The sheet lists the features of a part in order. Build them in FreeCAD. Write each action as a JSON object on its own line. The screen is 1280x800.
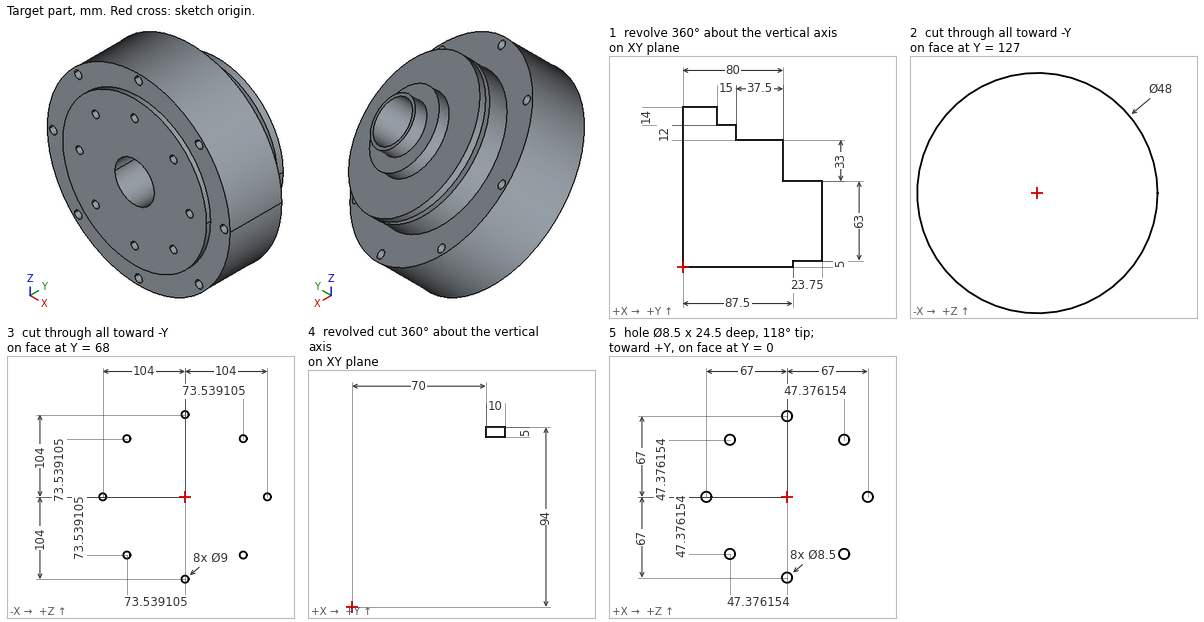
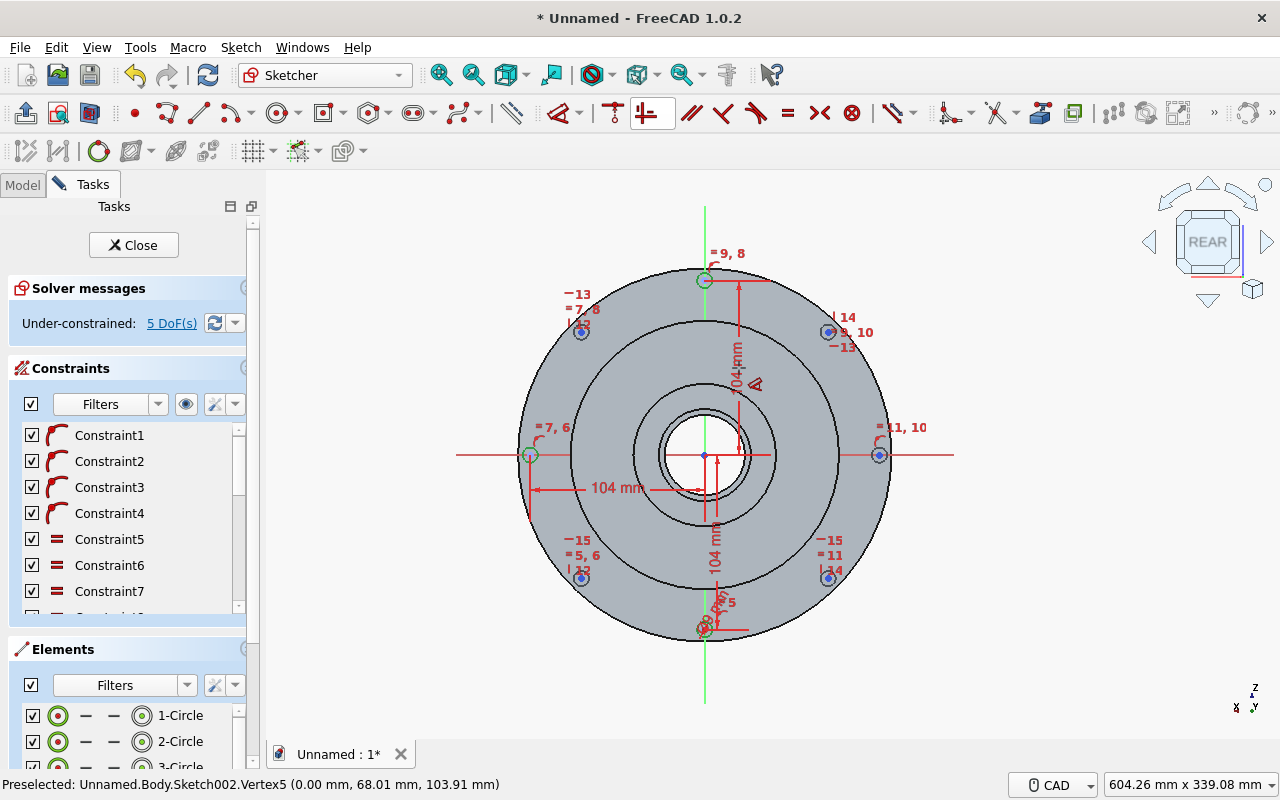
{"action": "left_click", "coordinate": [879, 455]}
{"action": "left_click", "coordinate": [792, 489]}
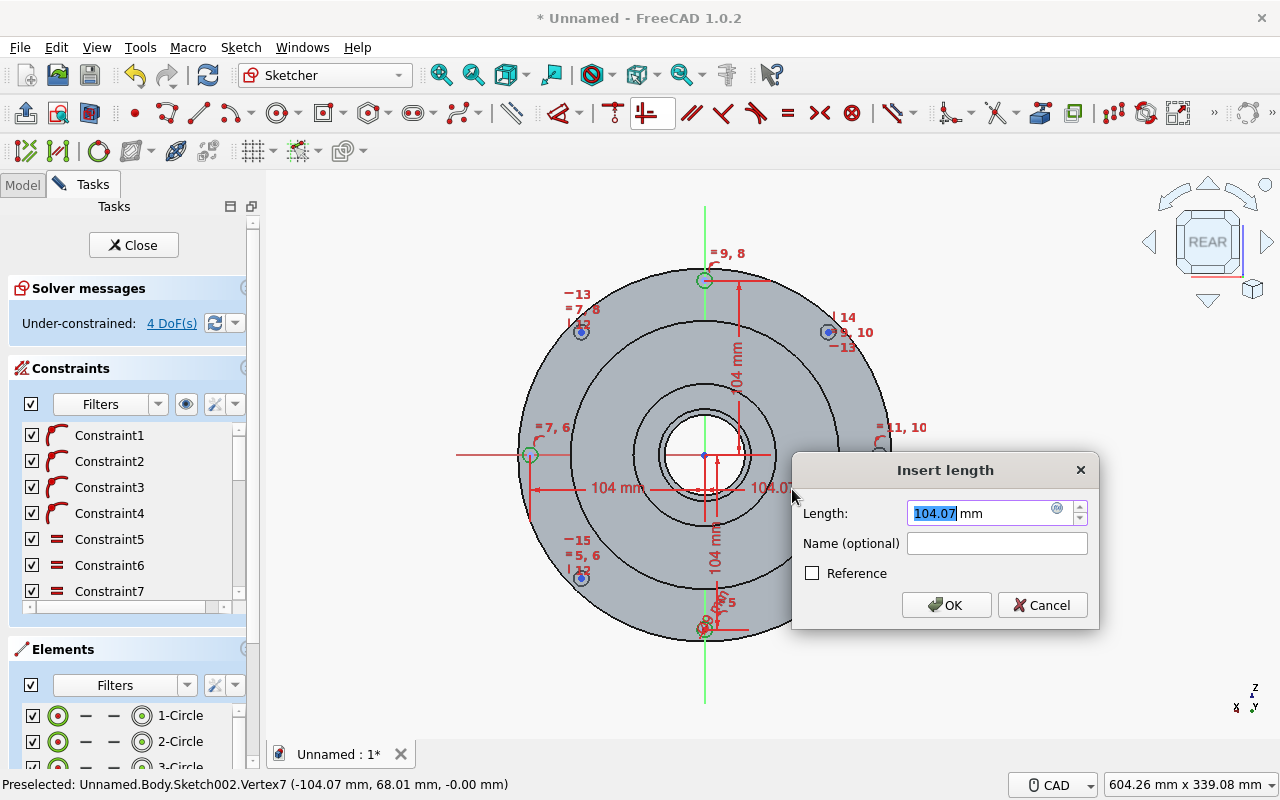
{"action": "type", "text": "104"}
{"action": "key", "text": "Return"}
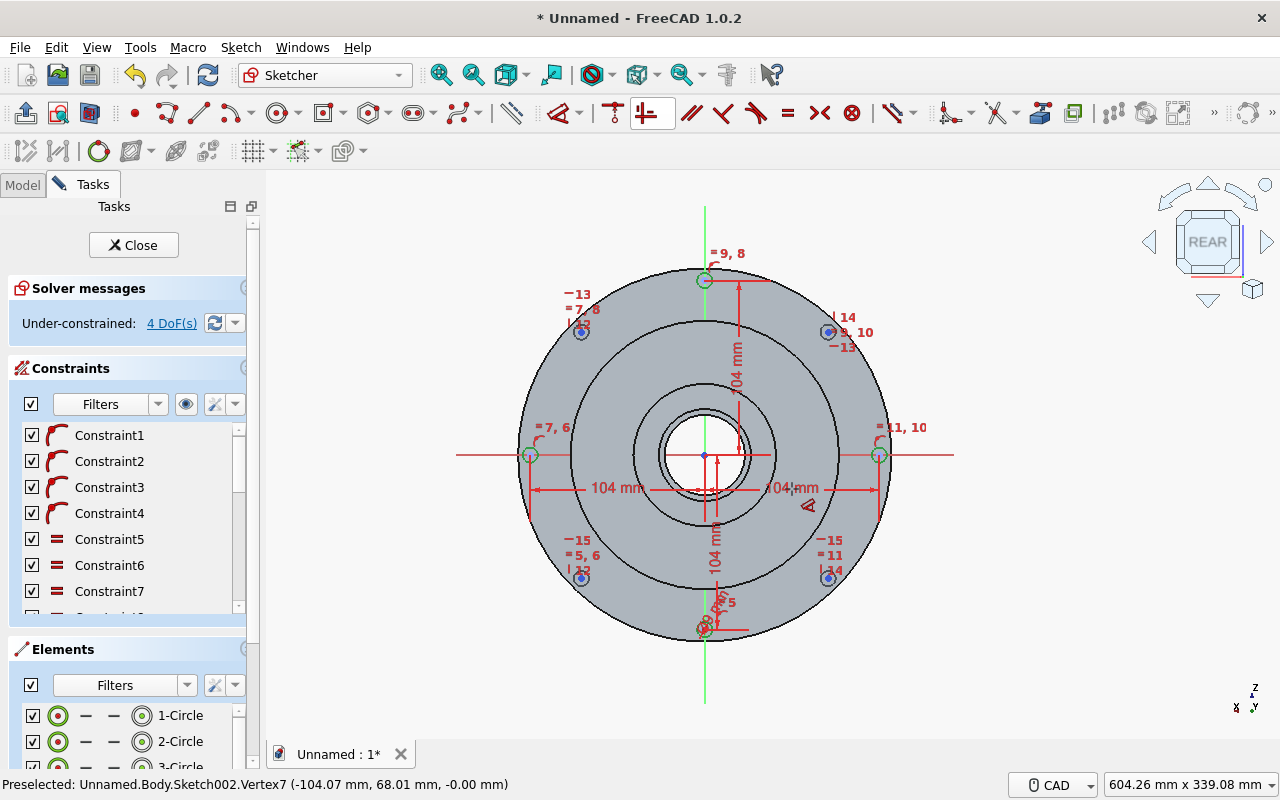
{"action": "left_click", "coordinate": [581, 579]}
{"action": "left_click", "coordinate": [643, 613]}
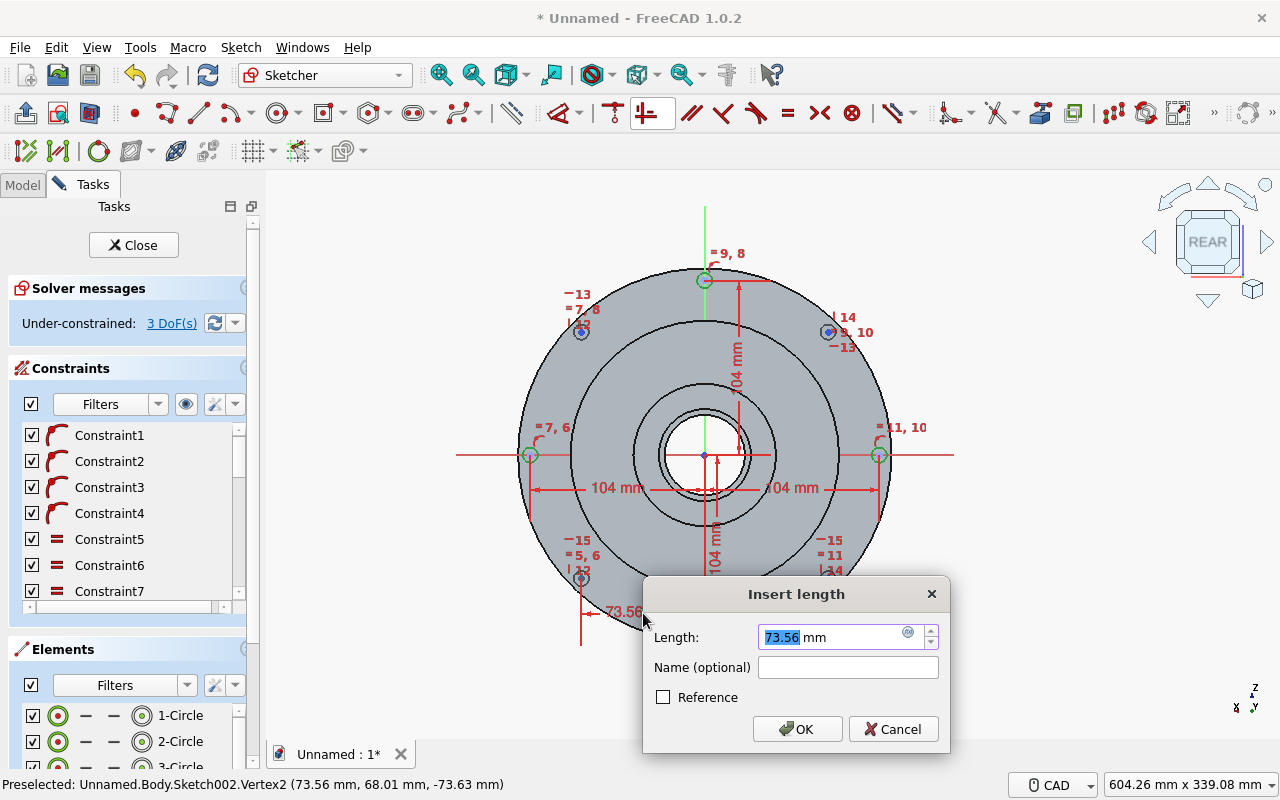
{"action": "type", "text": "73.539105"}
{"action": "key", "text": "Return"}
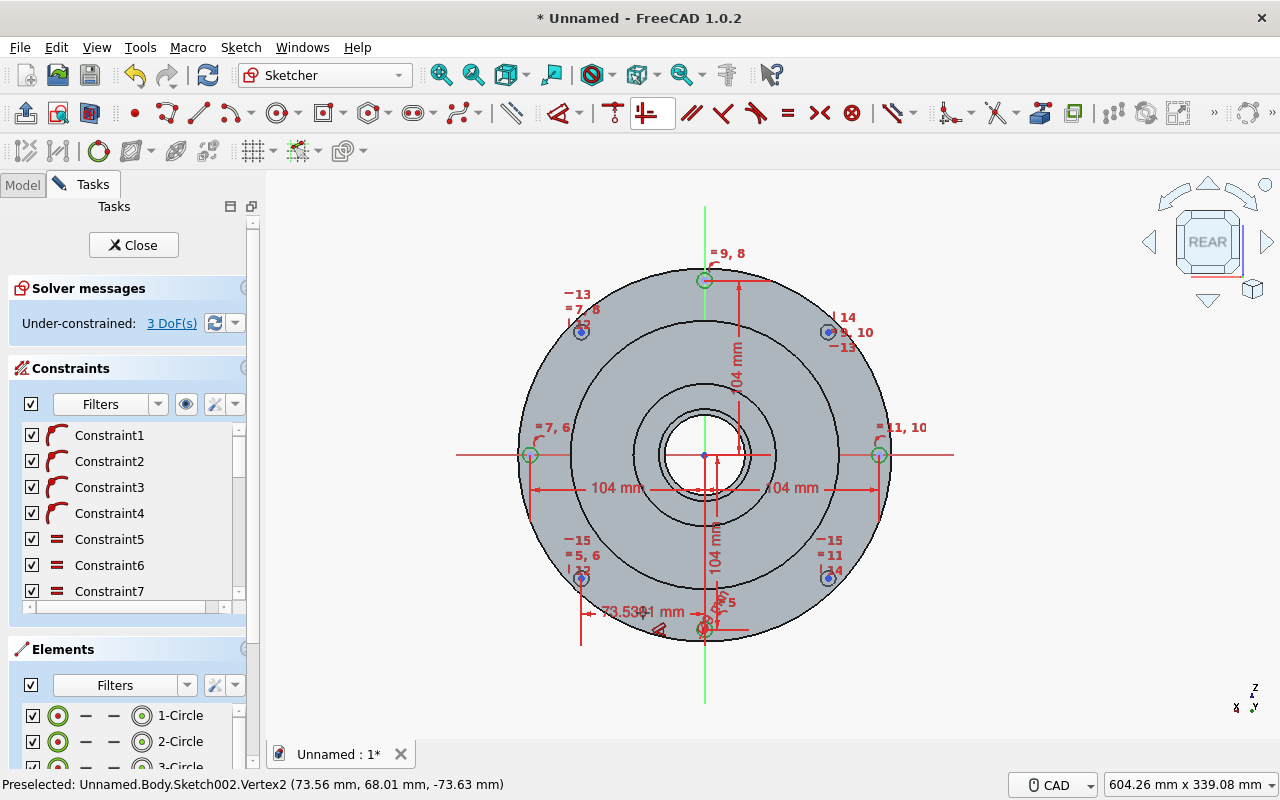
{"action": "left_click", "coordinate": [581, 579]}
{"action": "left_click", "coordinate": [547, 517]}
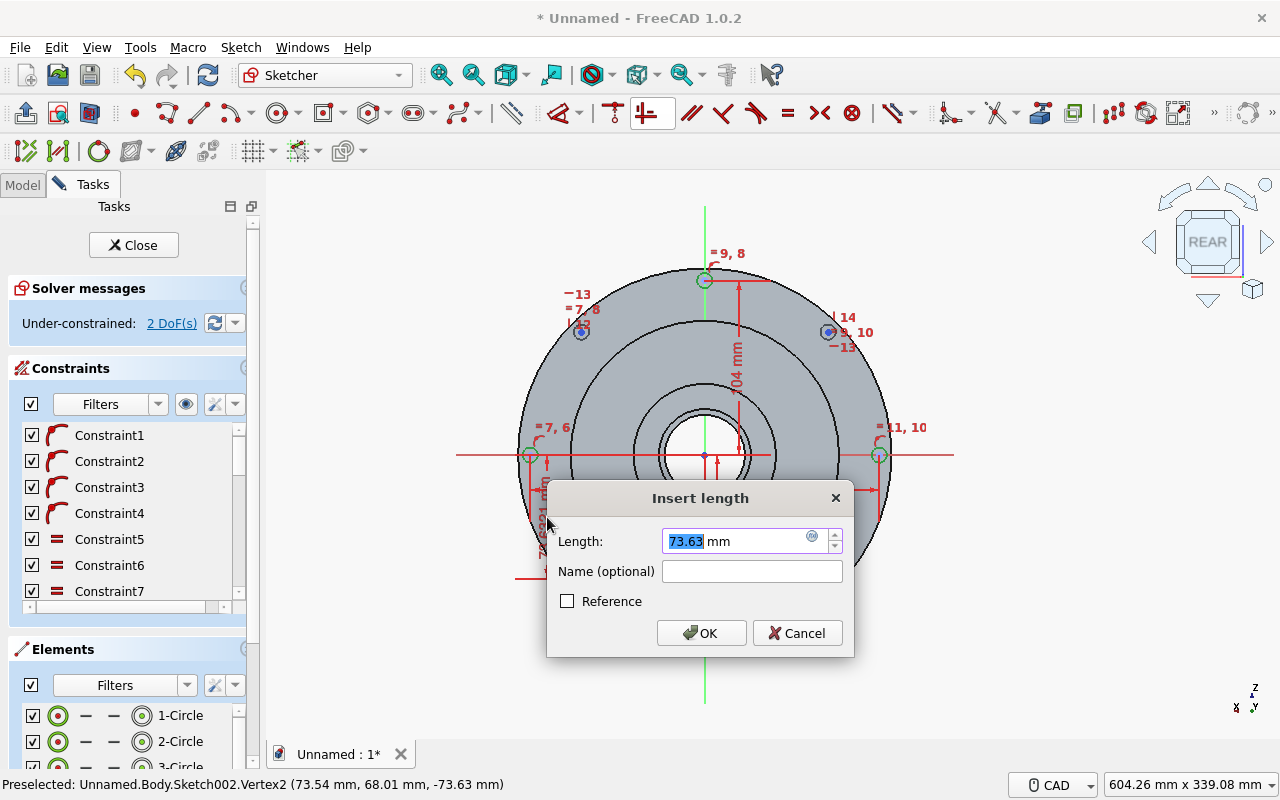
{"action": "type", "text": "73.539105"}
{"action": "key", "text": "Return"}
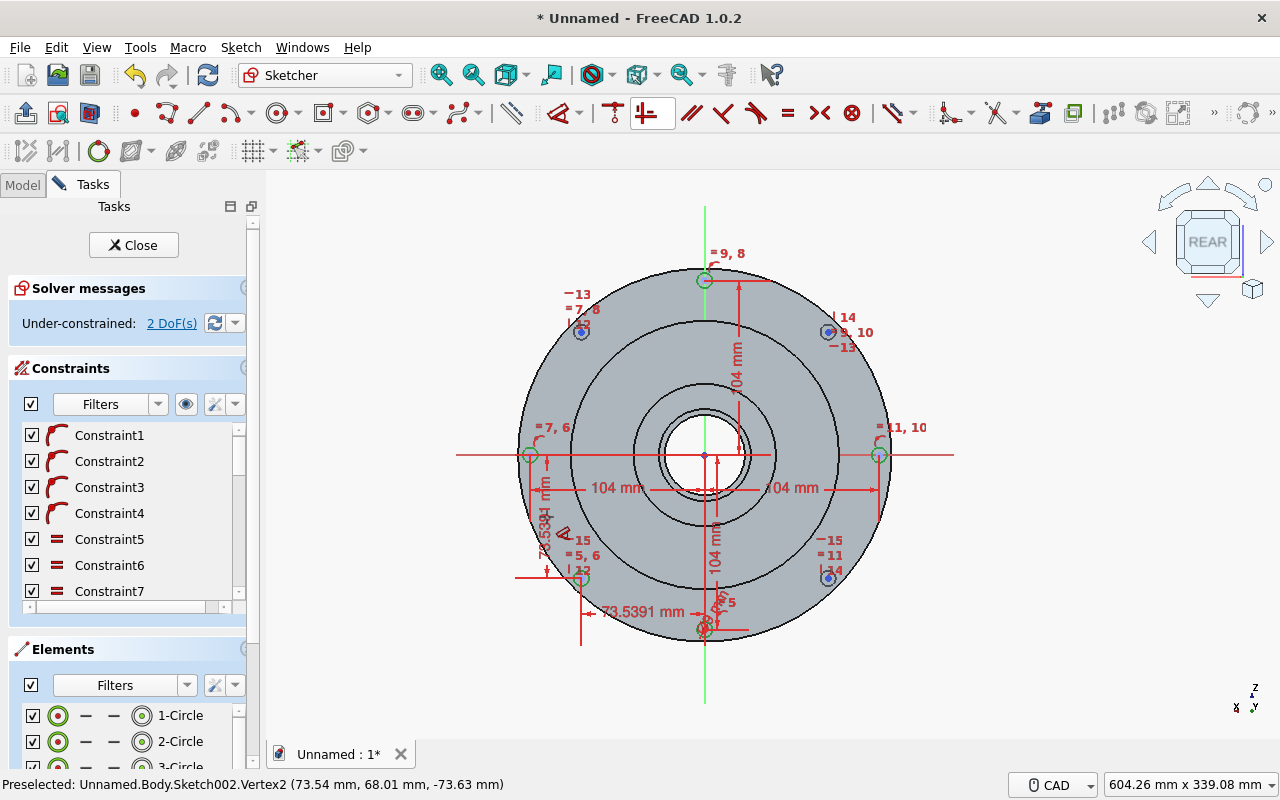
{"action": "left_click", "coordinate": [581, 332]}
{"action": "left_click", "coordinate": [547, 394]}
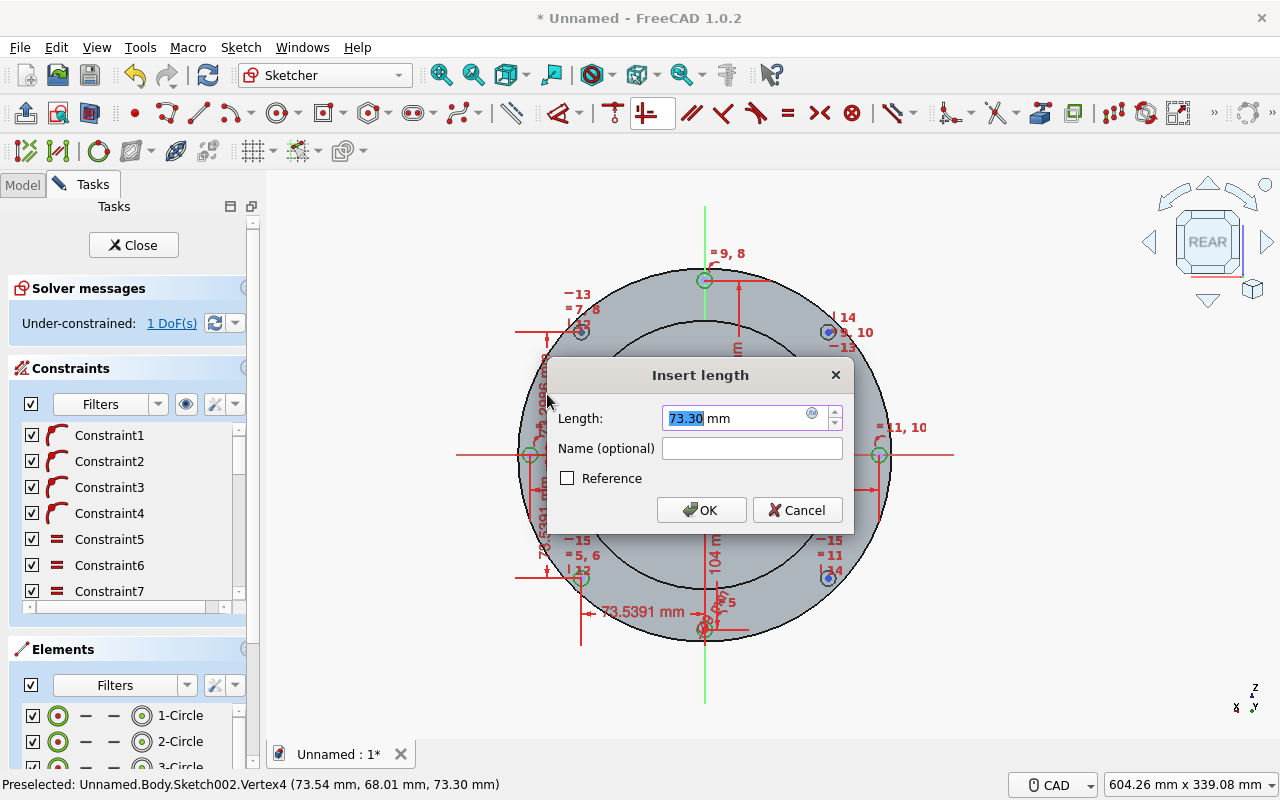
{"action": "type", "text": "73.539105"}
{"action": "key", "text": "Return"}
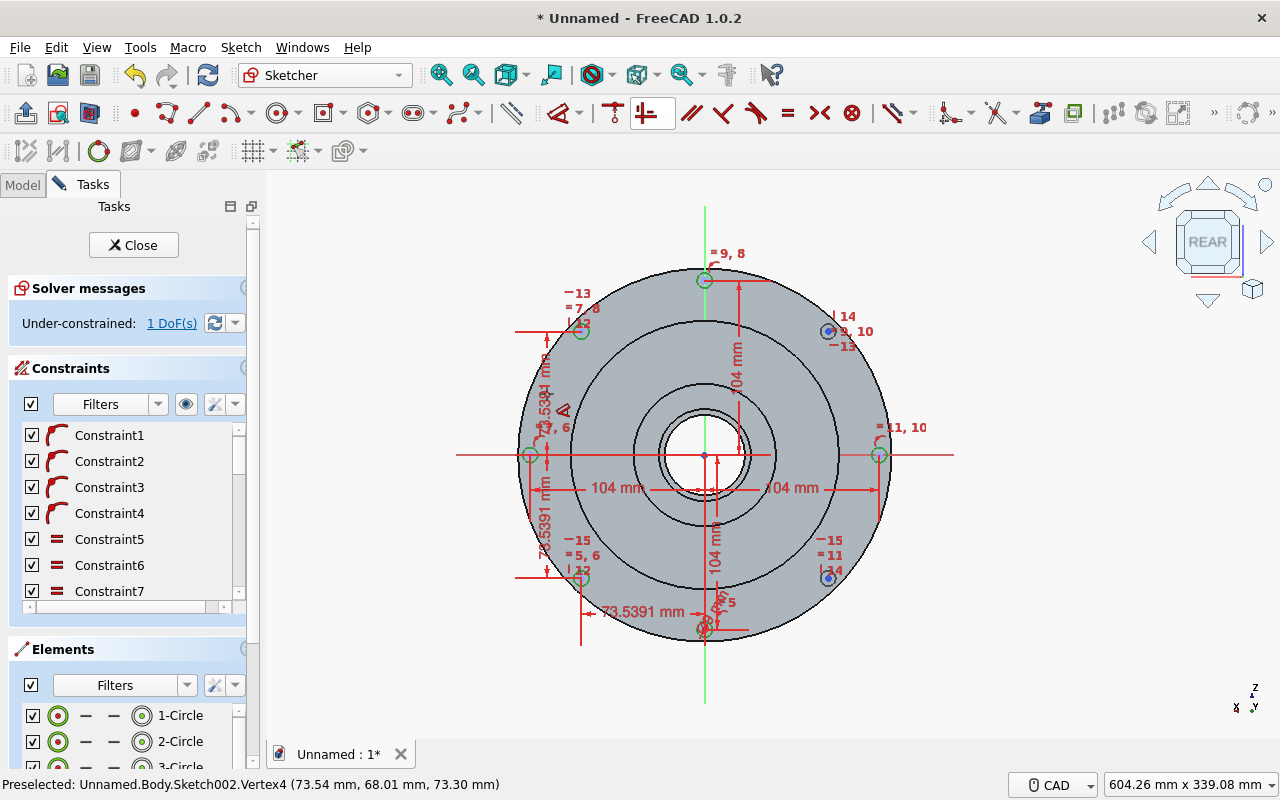
{"action": "left_click", "coordinate": [828, 332]}
{"action": "left_click", "coordinate": [766, 298]}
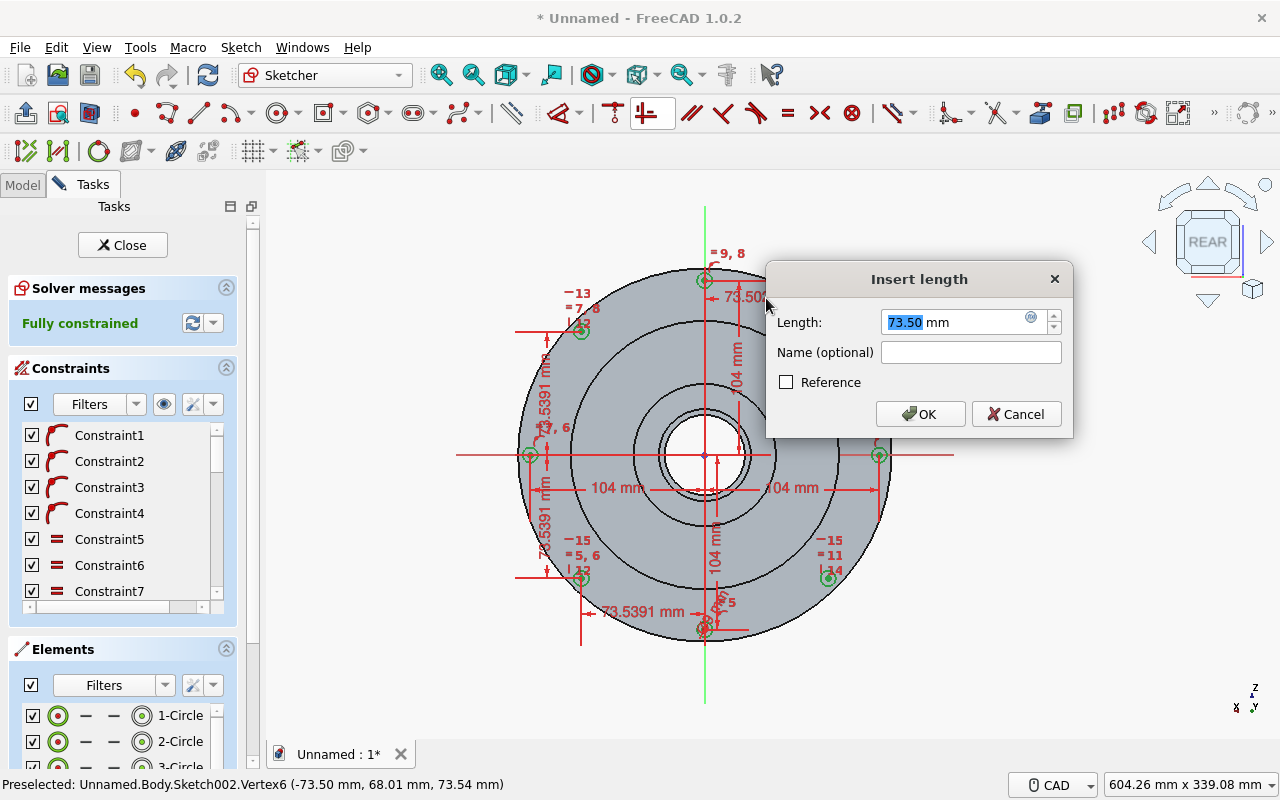
{"action": "type", "text": "73.539105"}
{"action": "key", "text": "Return"}
{"action": "key", "text": "Escape"}